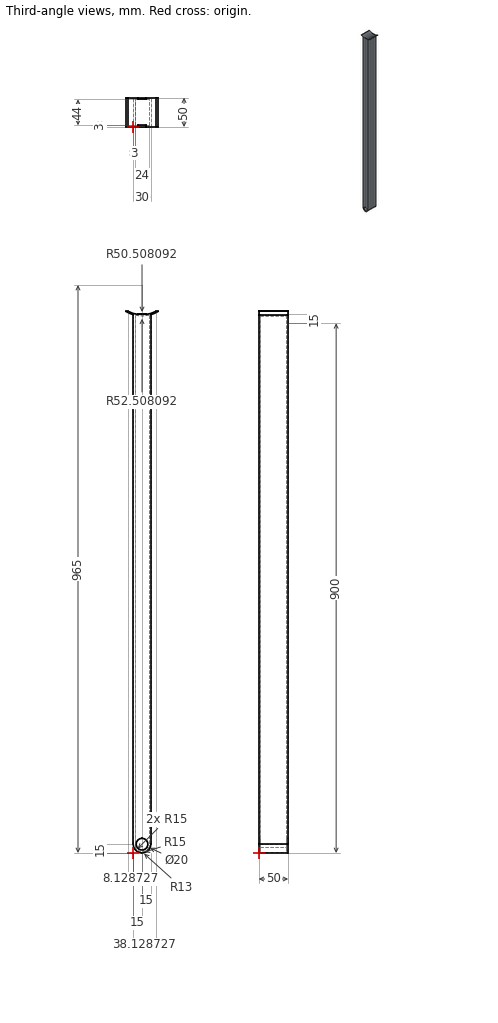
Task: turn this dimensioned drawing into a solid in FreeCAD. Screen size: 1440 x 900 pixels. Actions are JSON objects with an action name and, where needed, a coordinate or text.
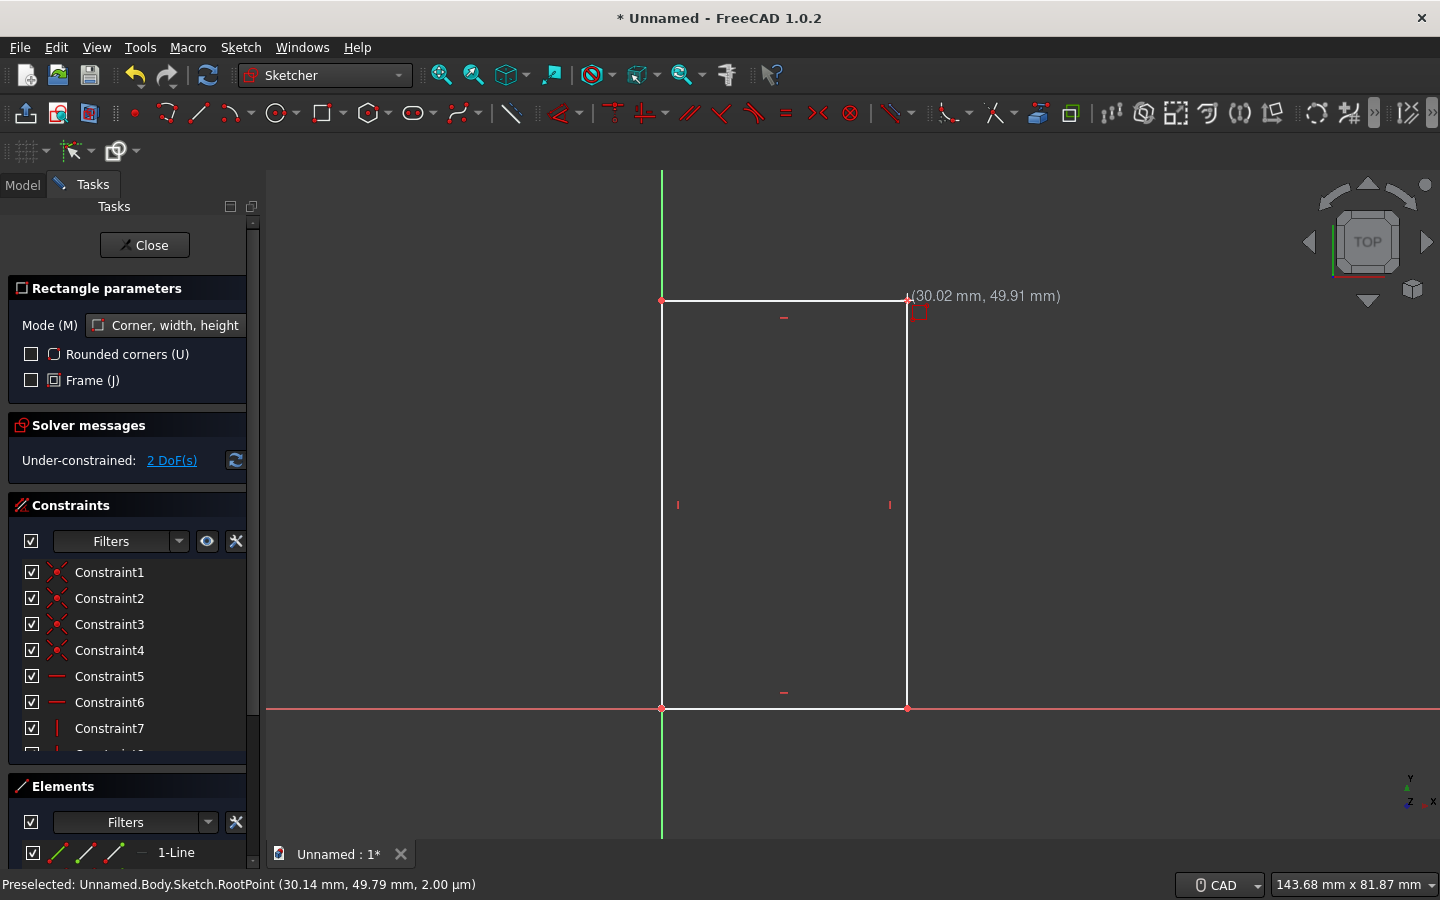
{"action": "left_click", "coordinate": [686, 325]}
{"action": "left_click", "coordinate": [882, 684]}
{"action": "key", "text": "Escape"}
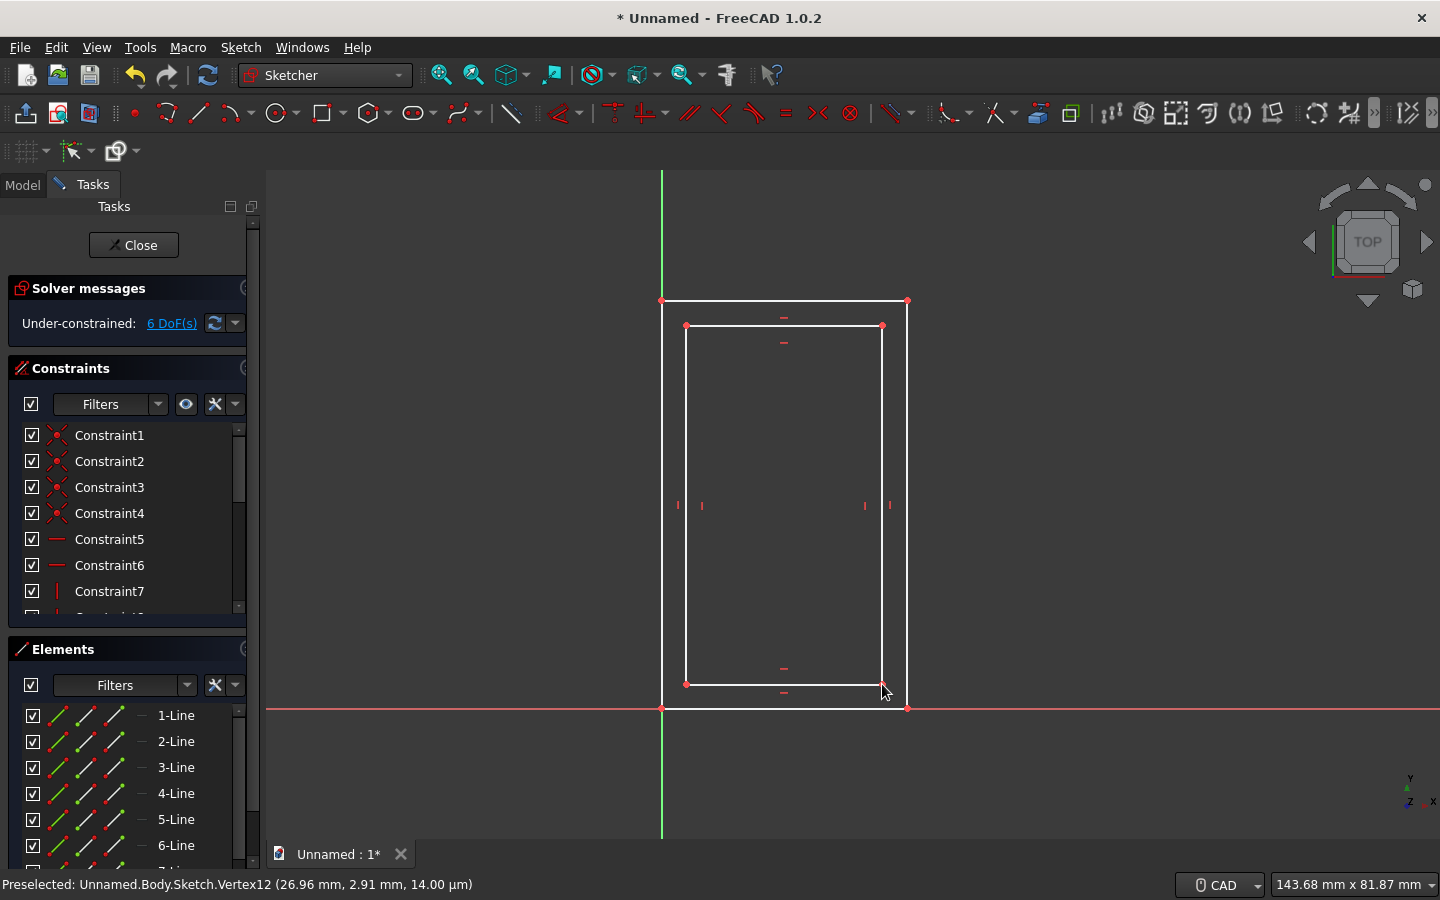
{"action": "left_click", "coordinate": [558, 114]}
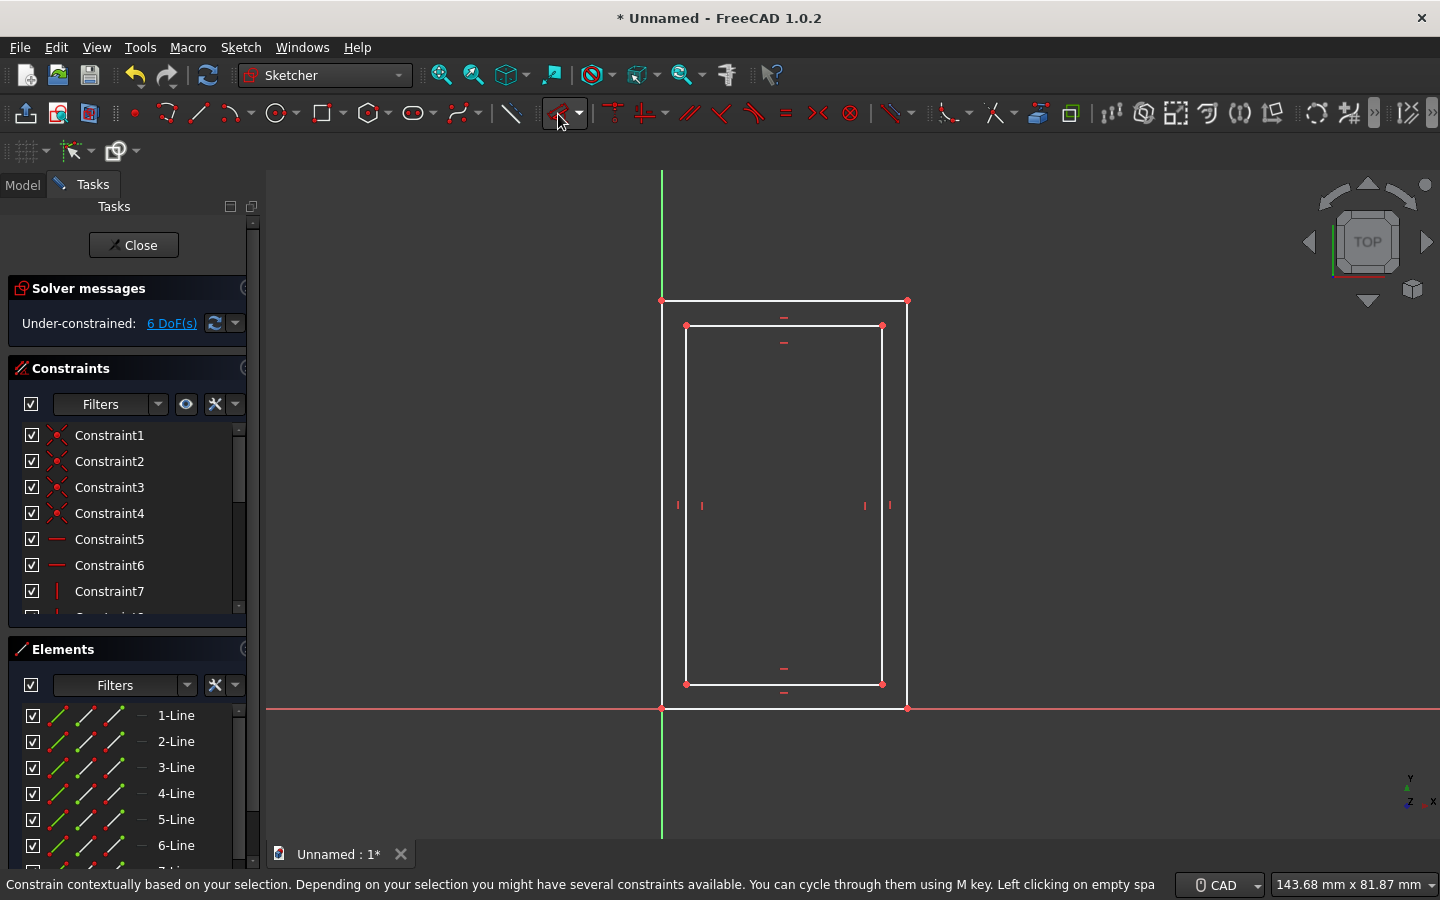
{"action": "left_click", "coordinate": [735, 709]}
{"action": "left_click", "coordinate": [784, 743]}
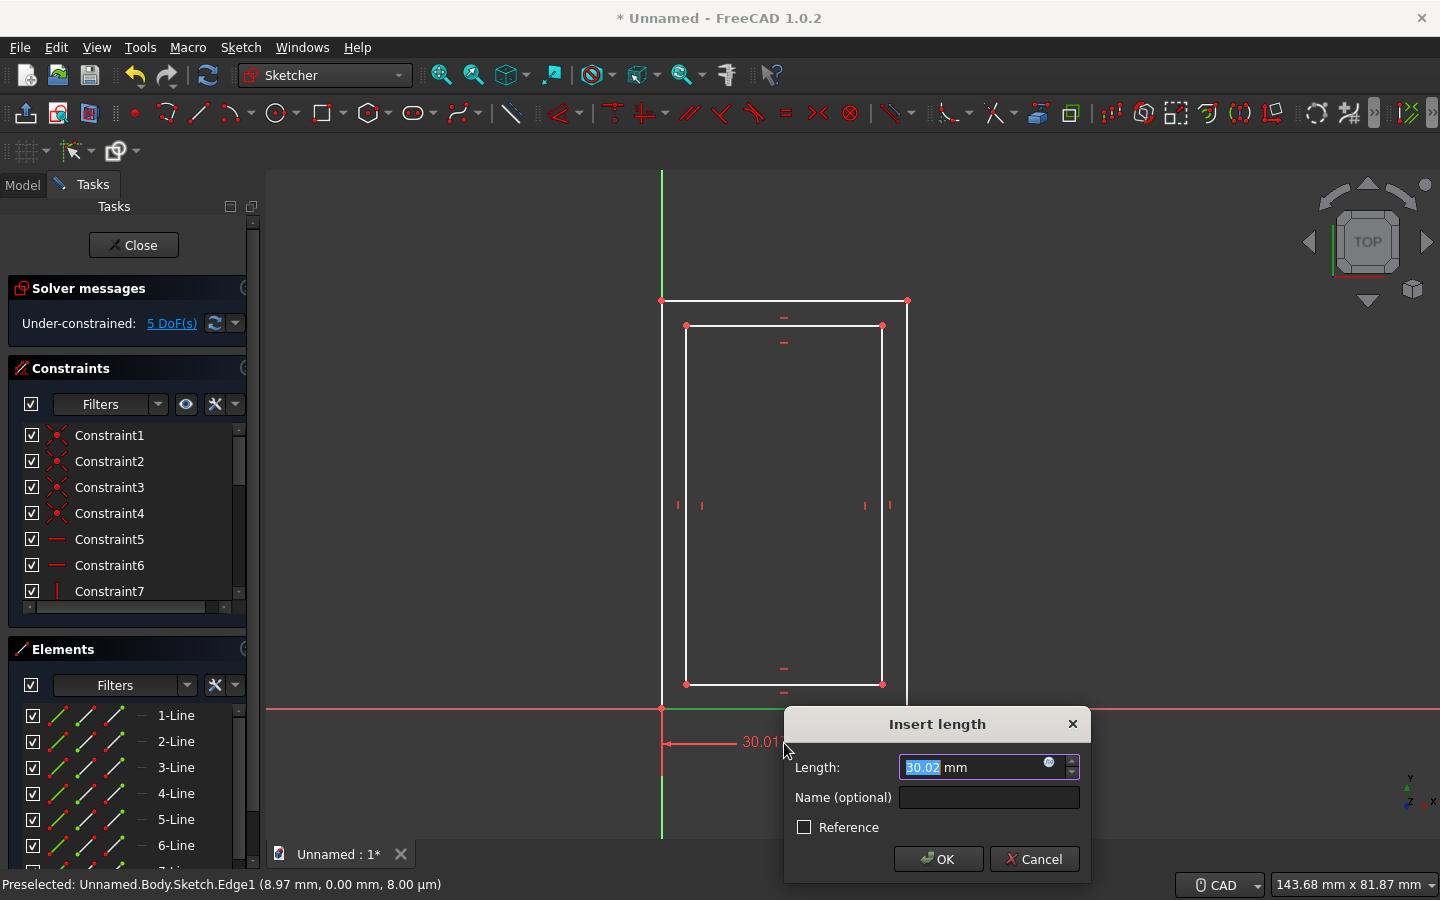
{"action": "type", "text": "30"}
{"action": "key", "text": "Return"}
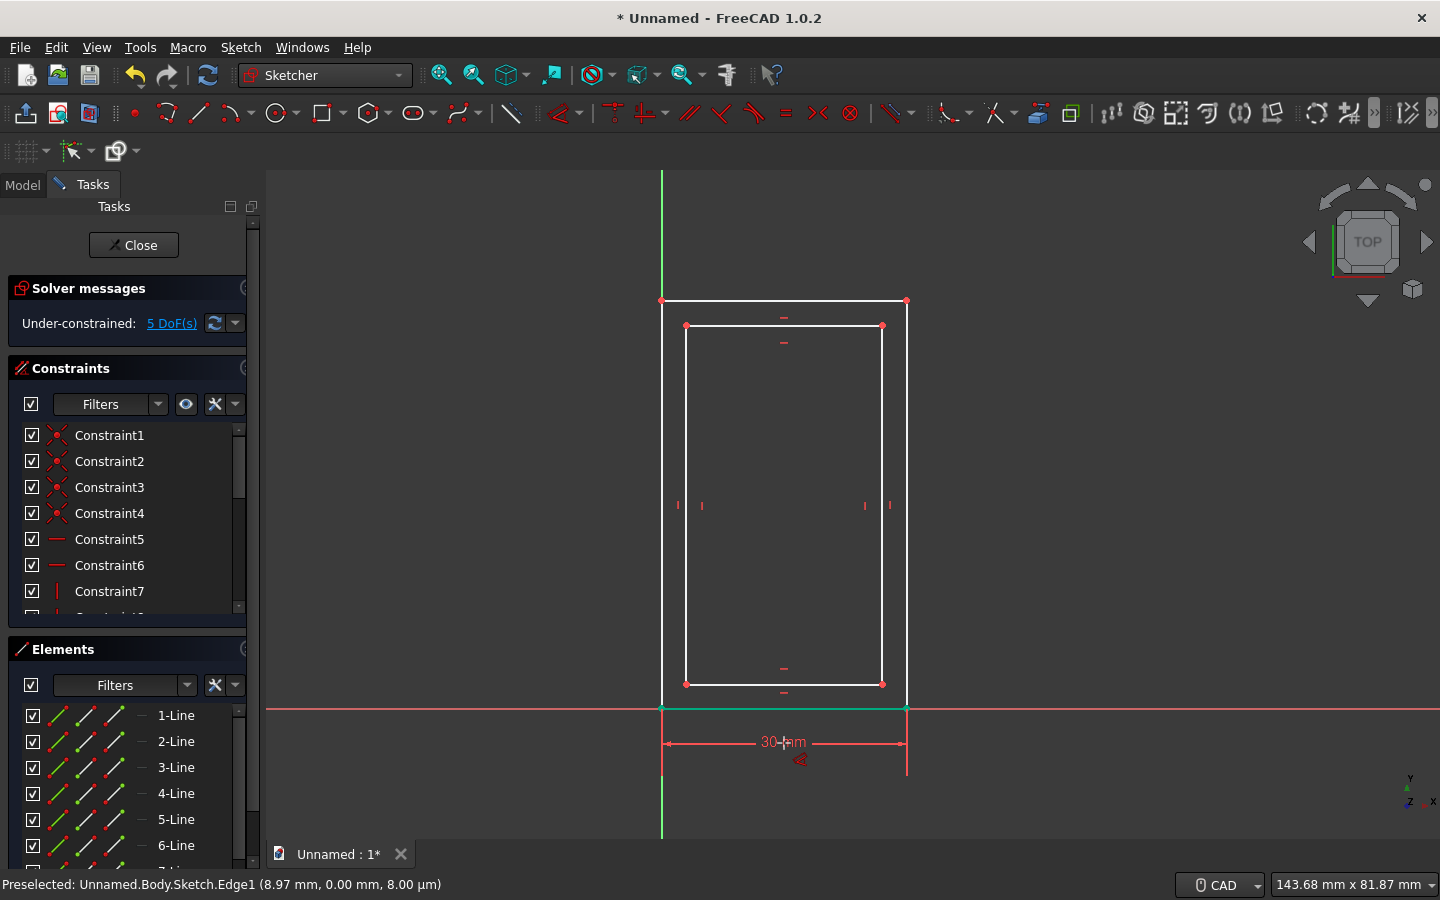
{"action": "left_click", "coordinate": [907, 586]}
{"action": "left_click", "coordinate": [941, 505]}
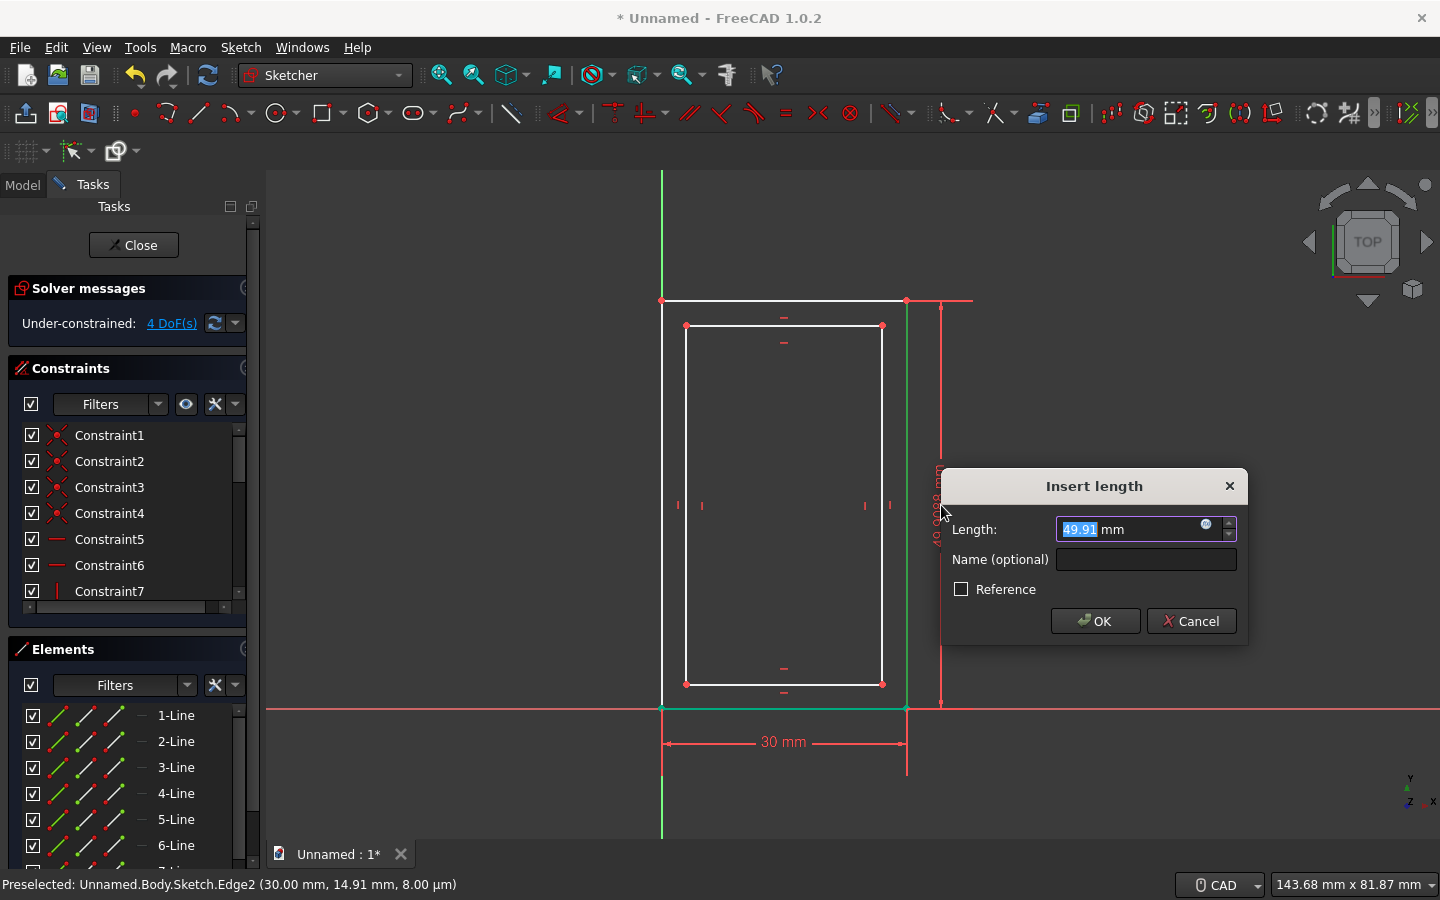
{"action": "type", "text": "50"}
{"action": "key", "text": "Return"}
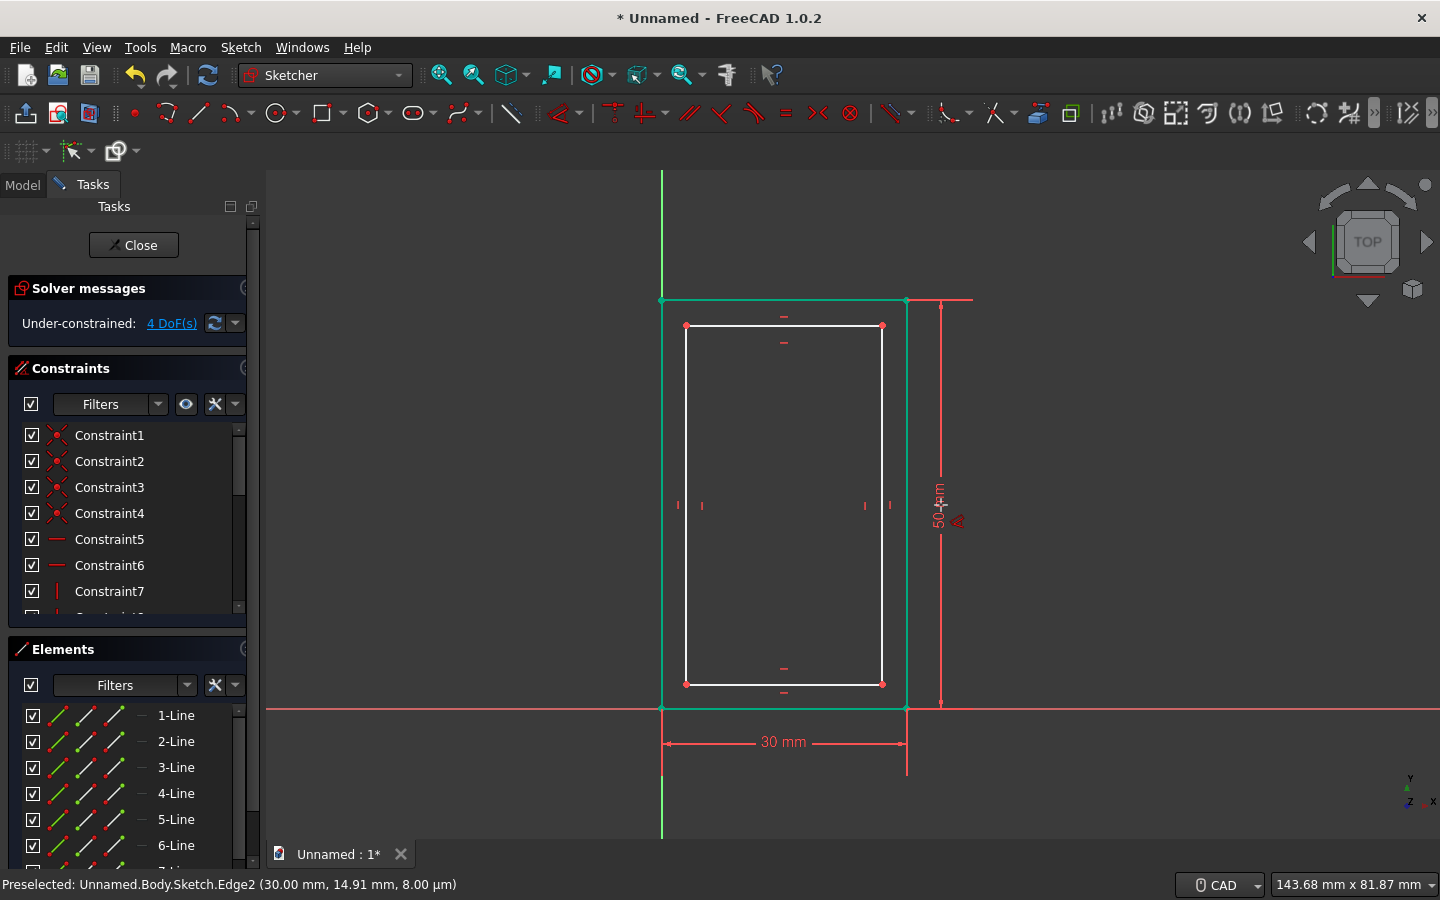
{"action": "left_click", "coordinate": [686, 434]}
{"action": "left_click", "coordinate": [720, 506]}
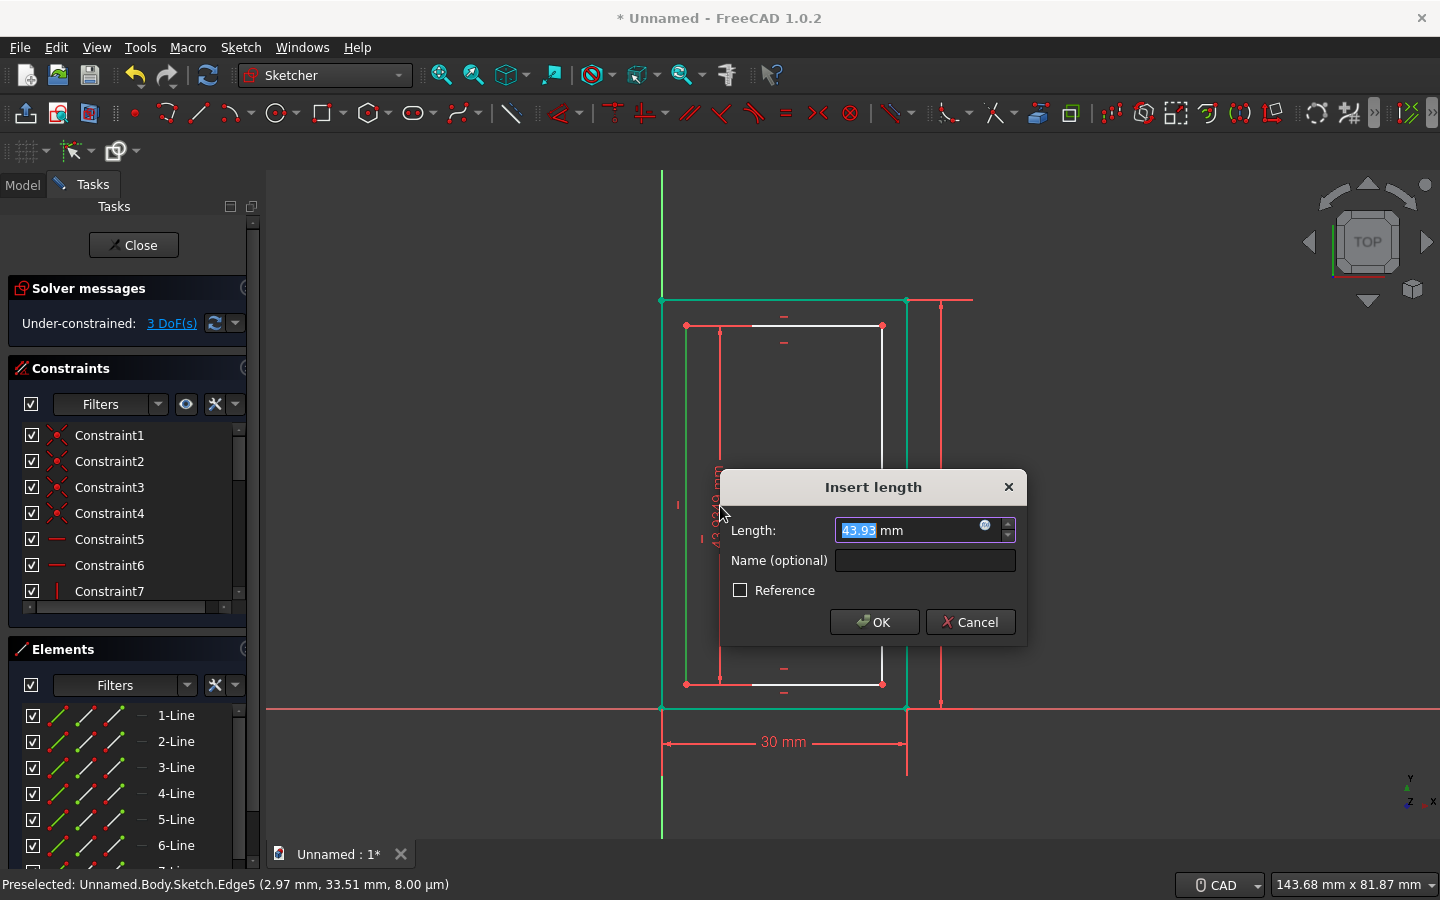
{"action": "type", "text": "44"}
{"action": "key", "text": "Return"}